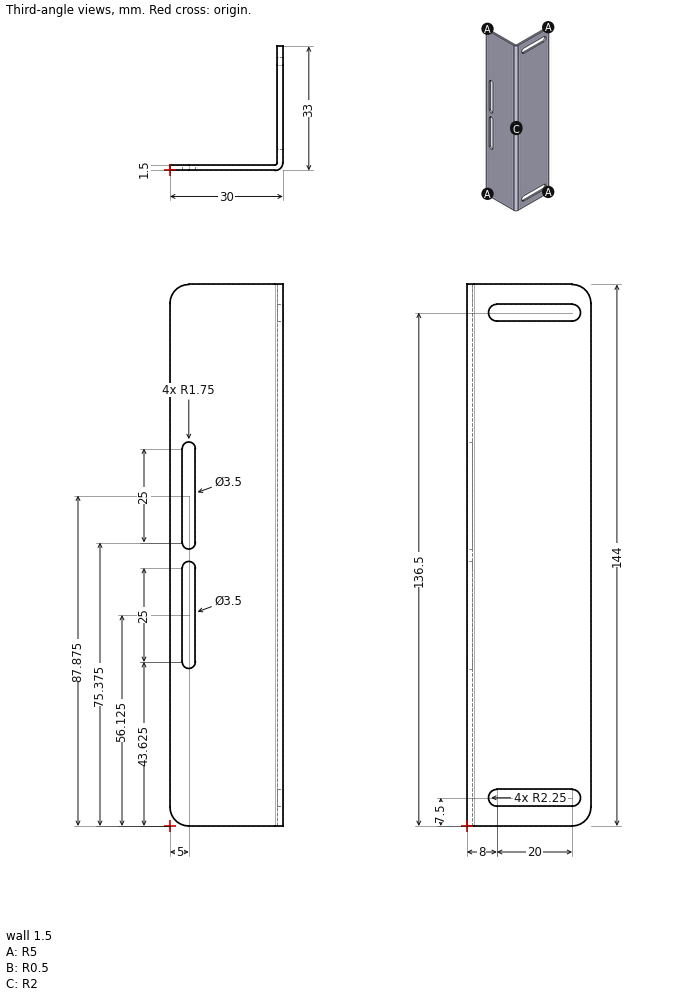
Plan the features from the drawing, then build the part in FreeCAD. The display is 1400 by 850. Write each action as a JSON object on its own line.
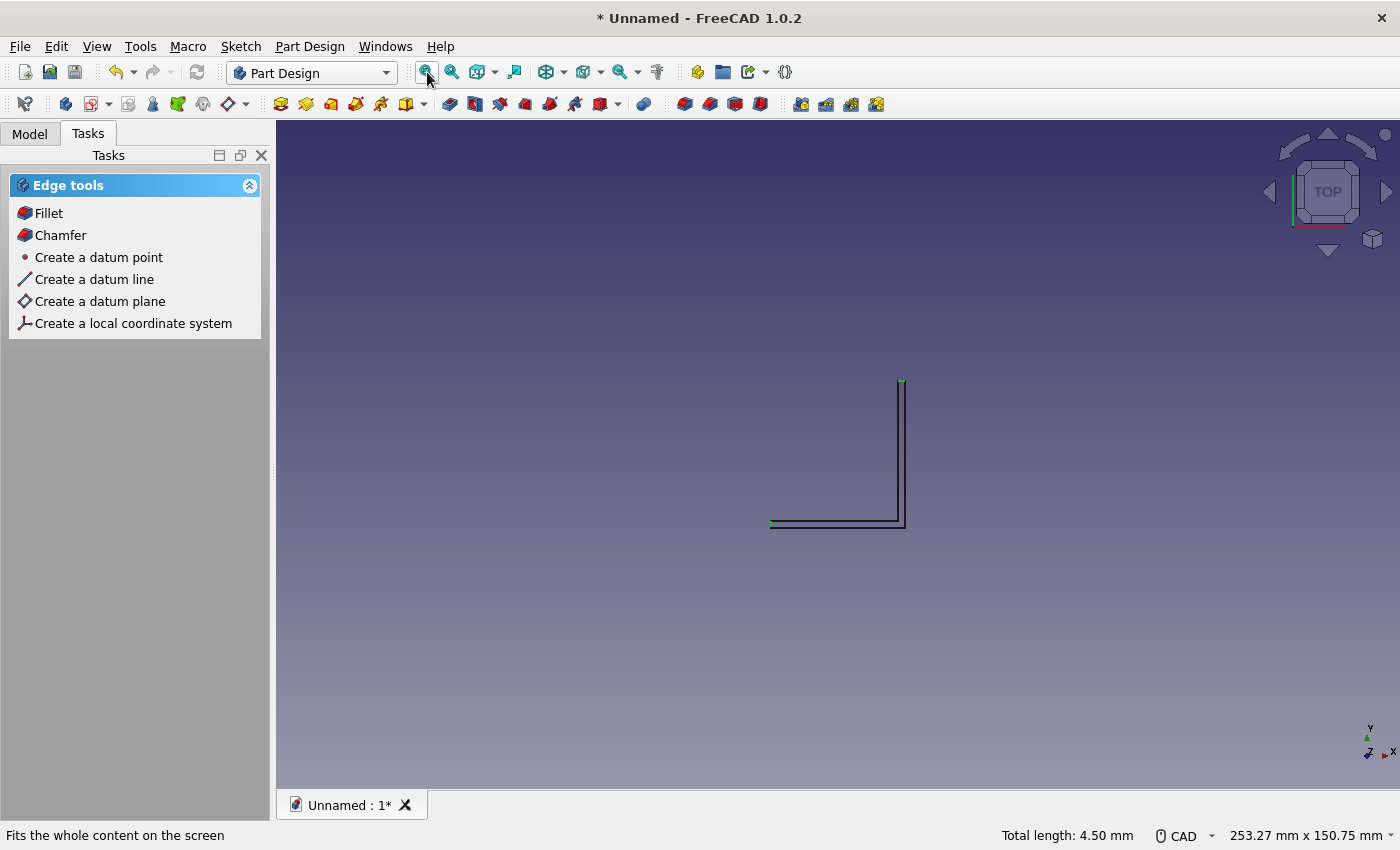
{"action": "key", "text": "1"}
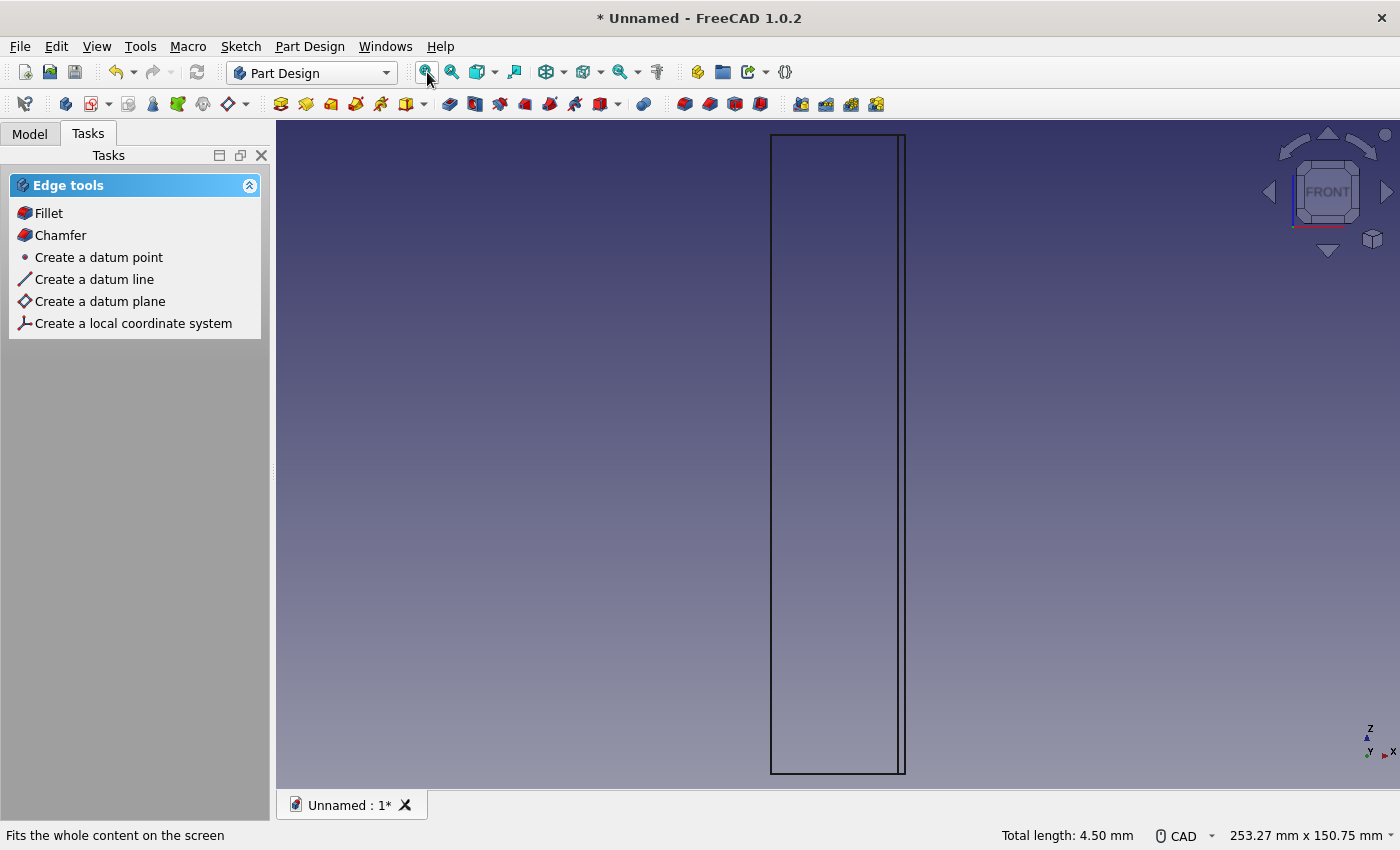
{"action": "key", "text": "3"}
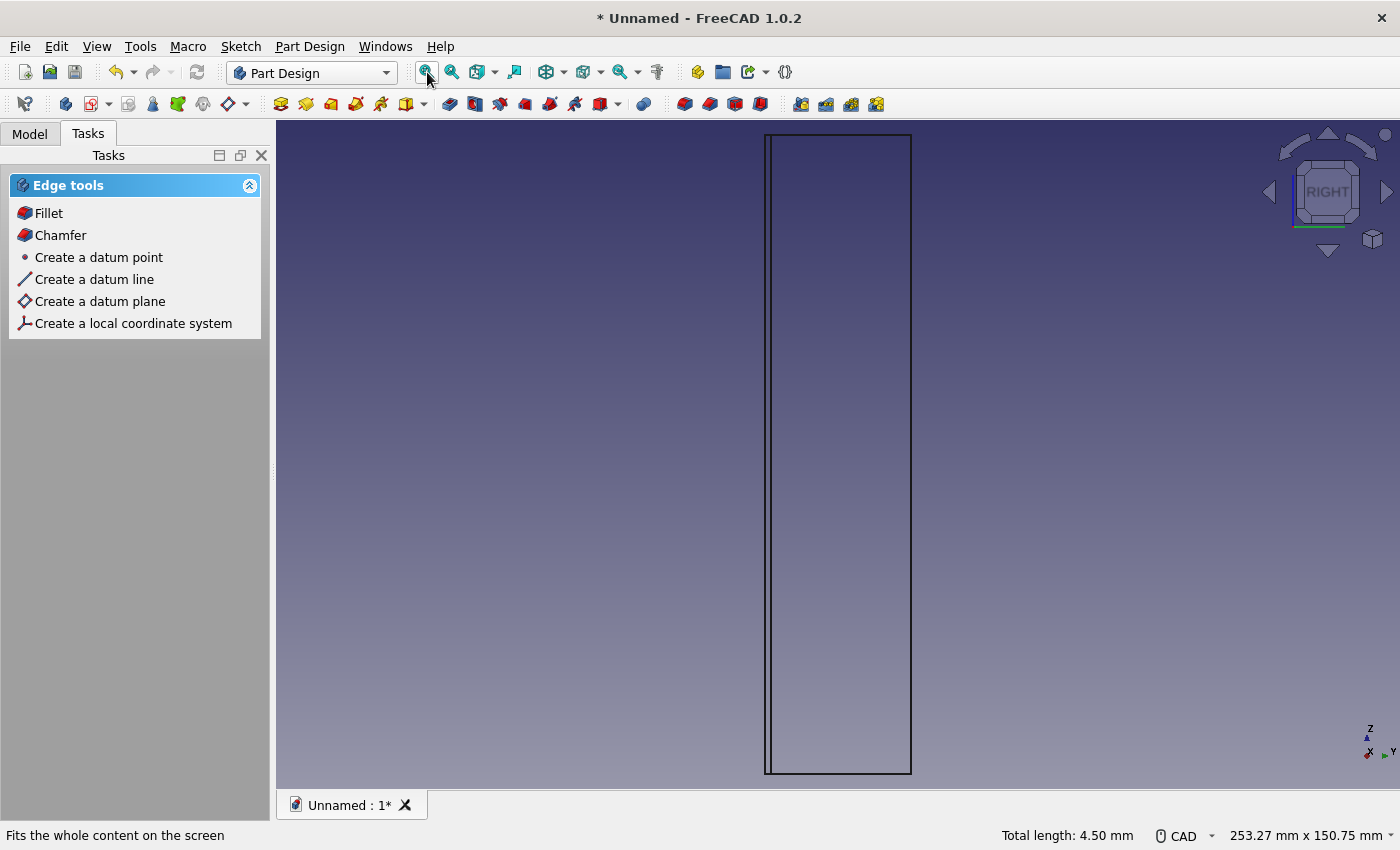
{"action": "key", "text": "5"}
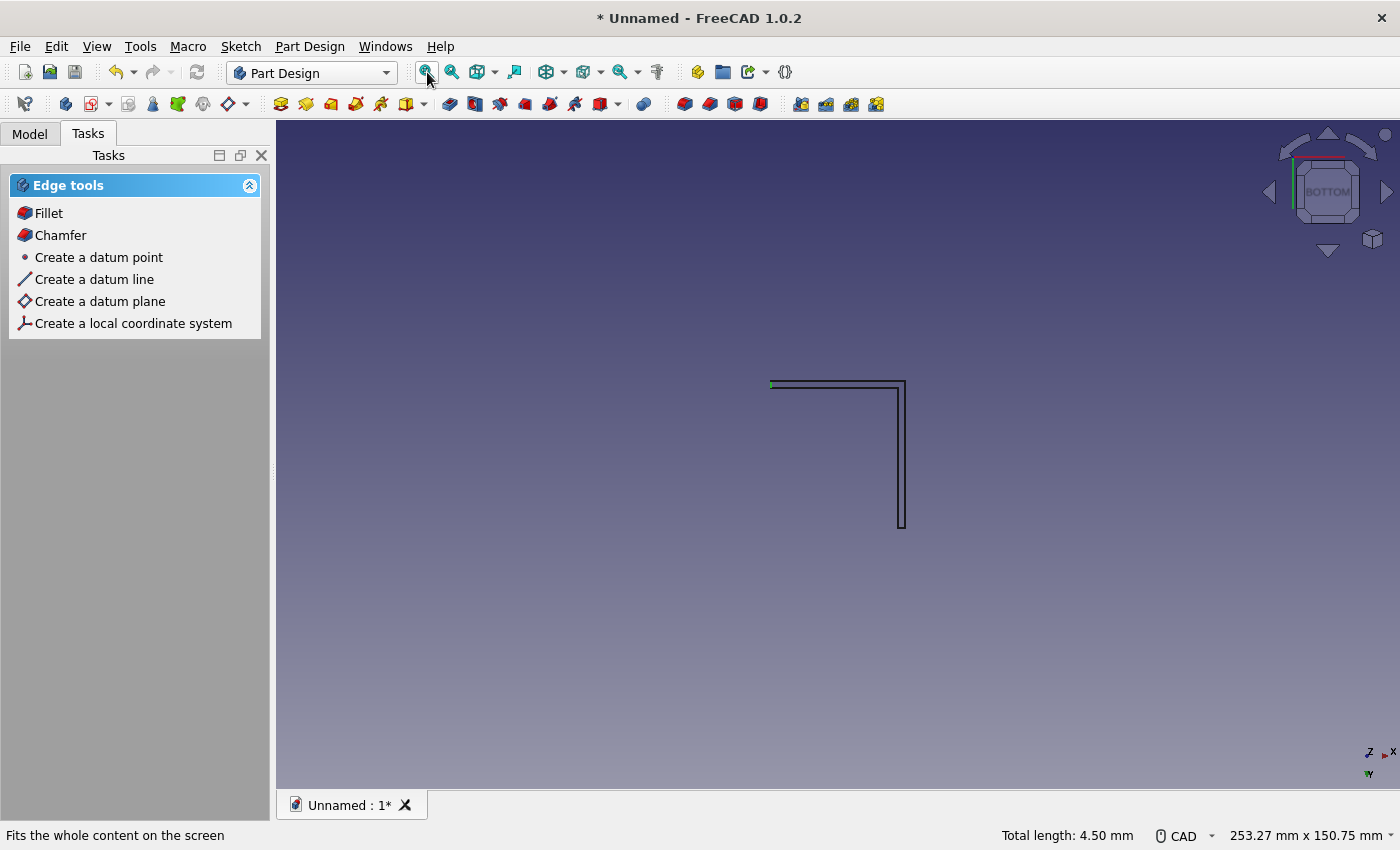
{"action": "left_click", "coordinate": [427, 72]}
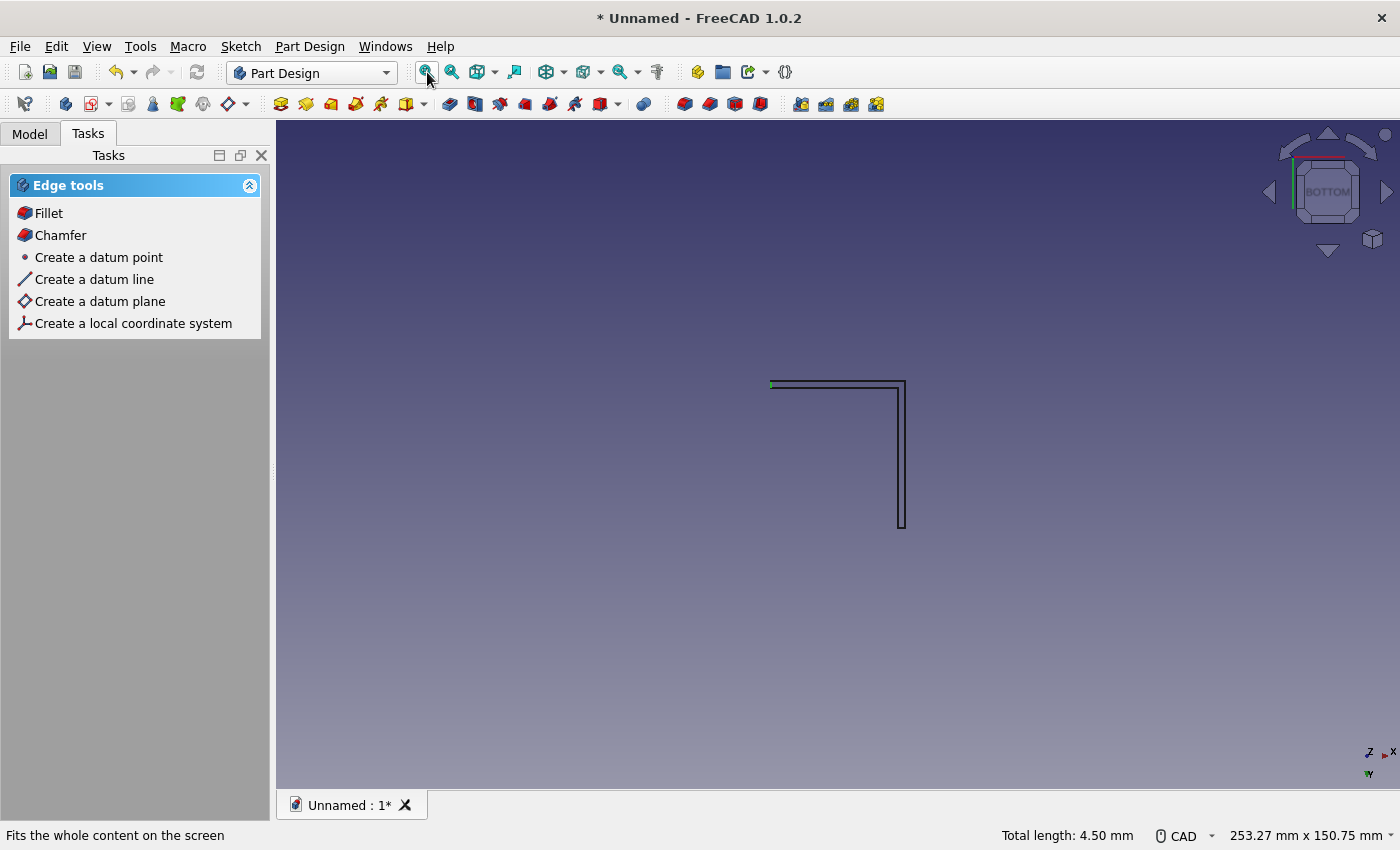
{"action": "scroll", "coordinate": [901, 527], "scroll_direction": "up", "scroll_amount": 9}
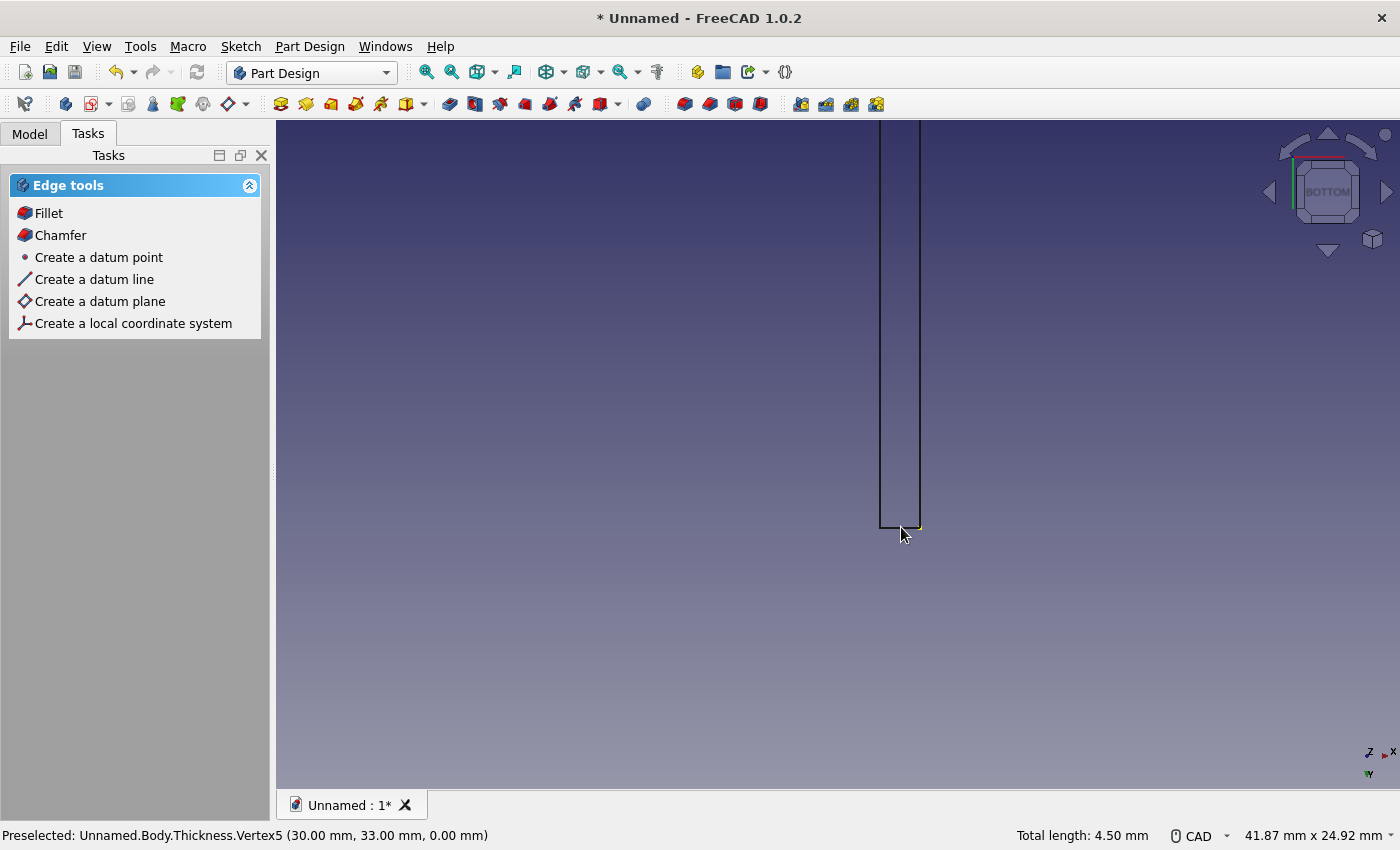
{"action": "left_click", "coordinate": [900, 527], "text": "ctrl"}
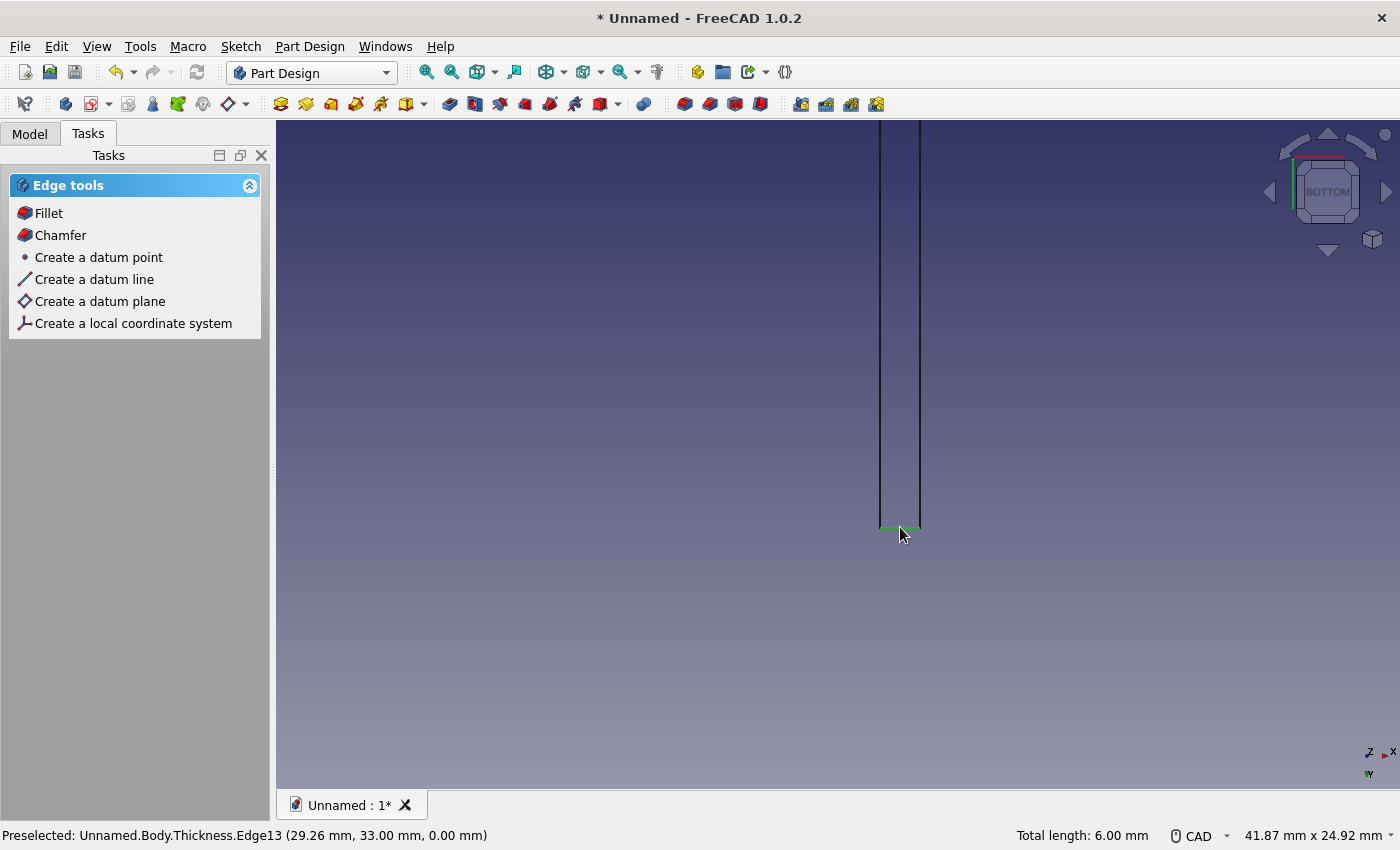
{"action": "key", "text": "v 1"}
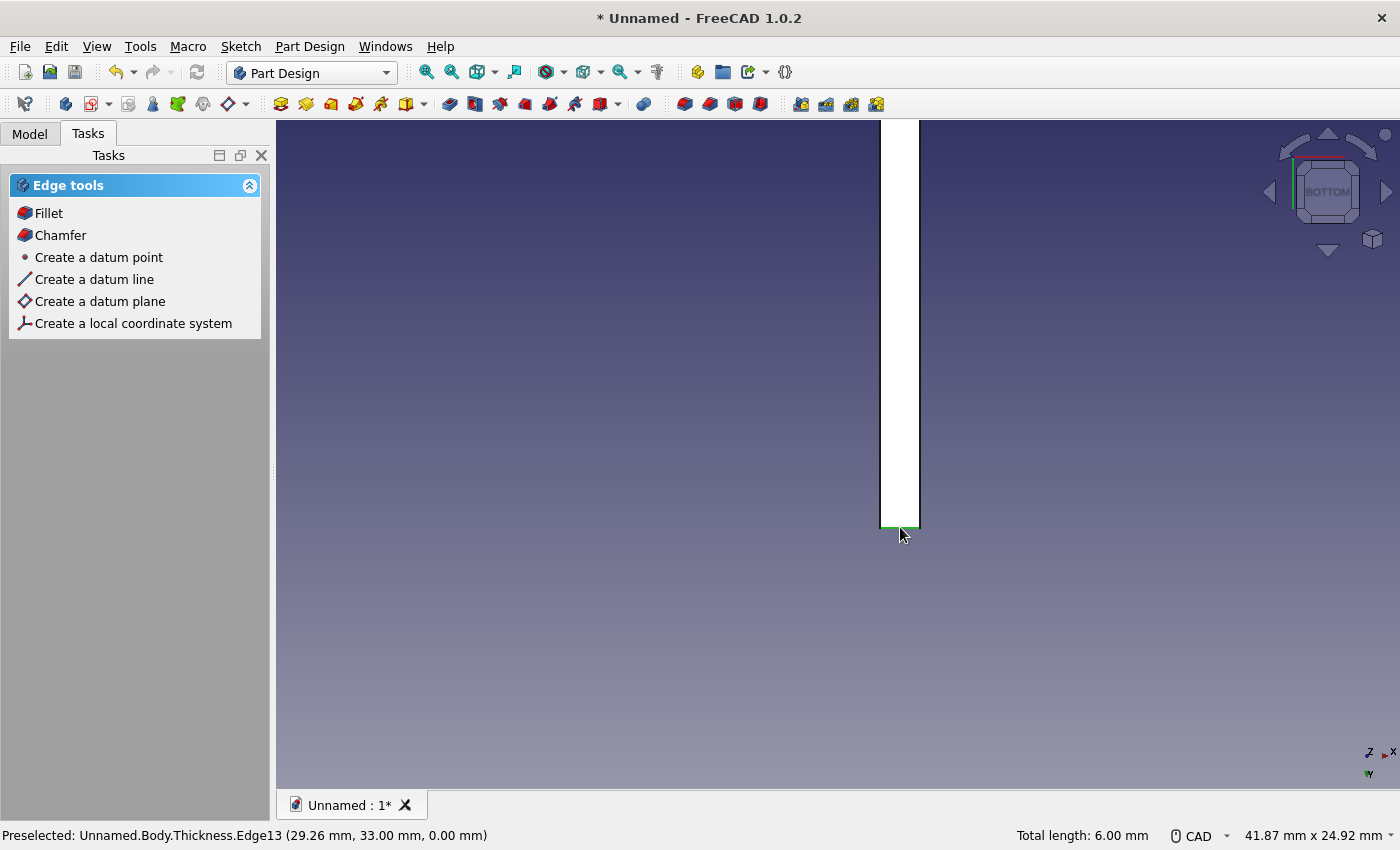
{"action": "left_click", "coordinate": [685, 104]}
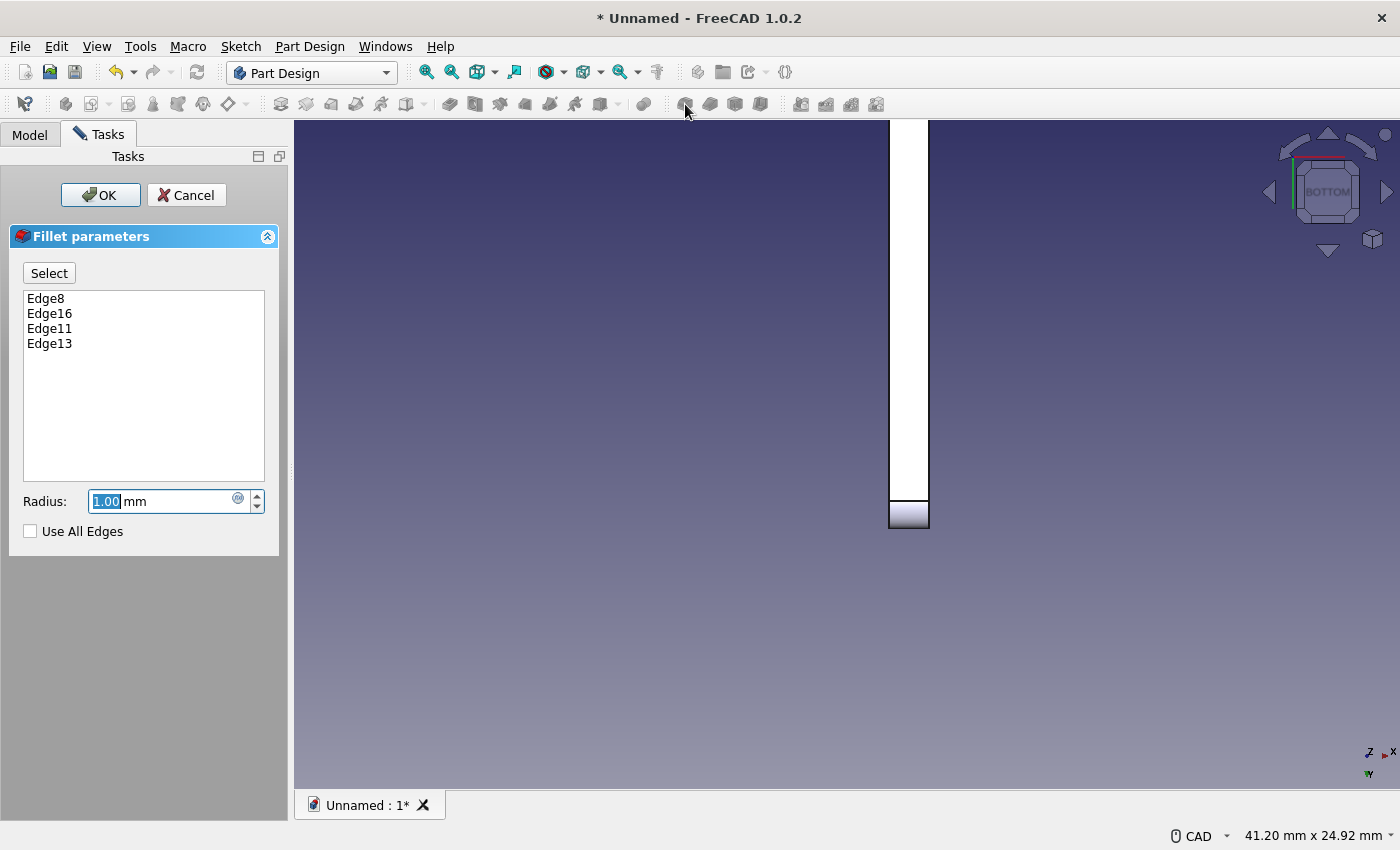
{"action": "type", "text": "5"}
{"action": "key", "text": "Tab"}